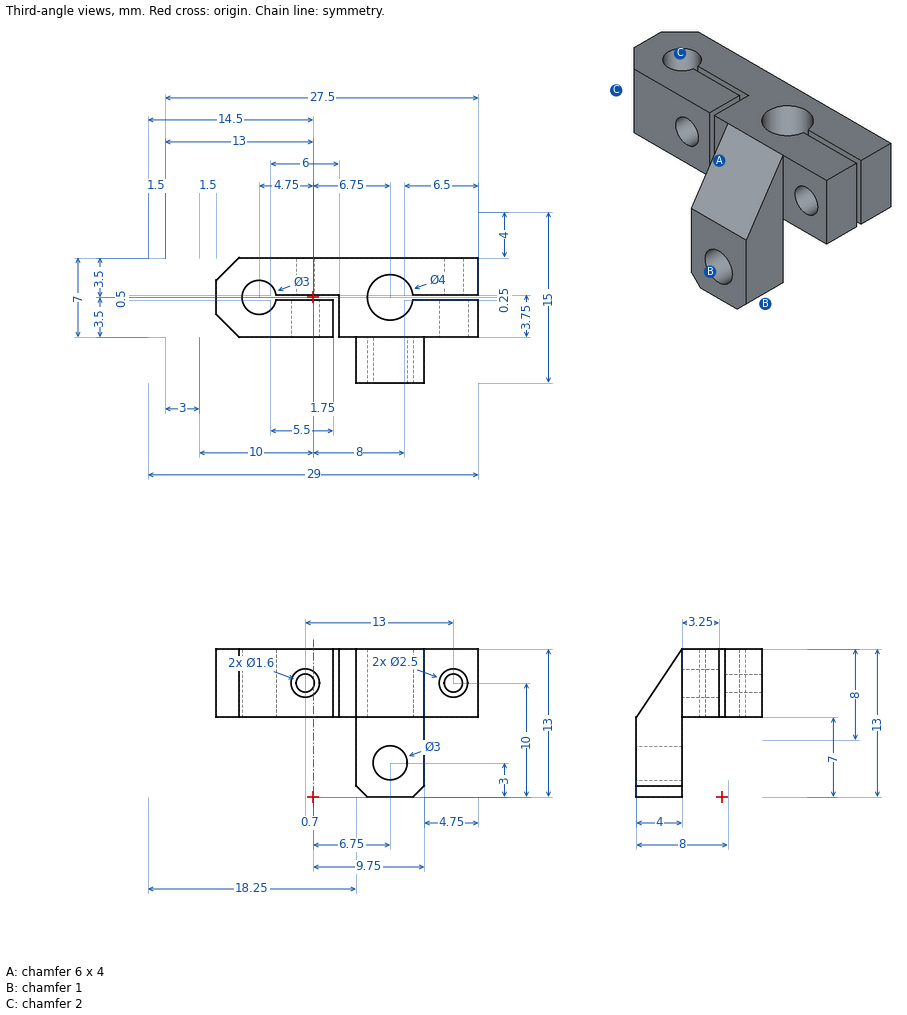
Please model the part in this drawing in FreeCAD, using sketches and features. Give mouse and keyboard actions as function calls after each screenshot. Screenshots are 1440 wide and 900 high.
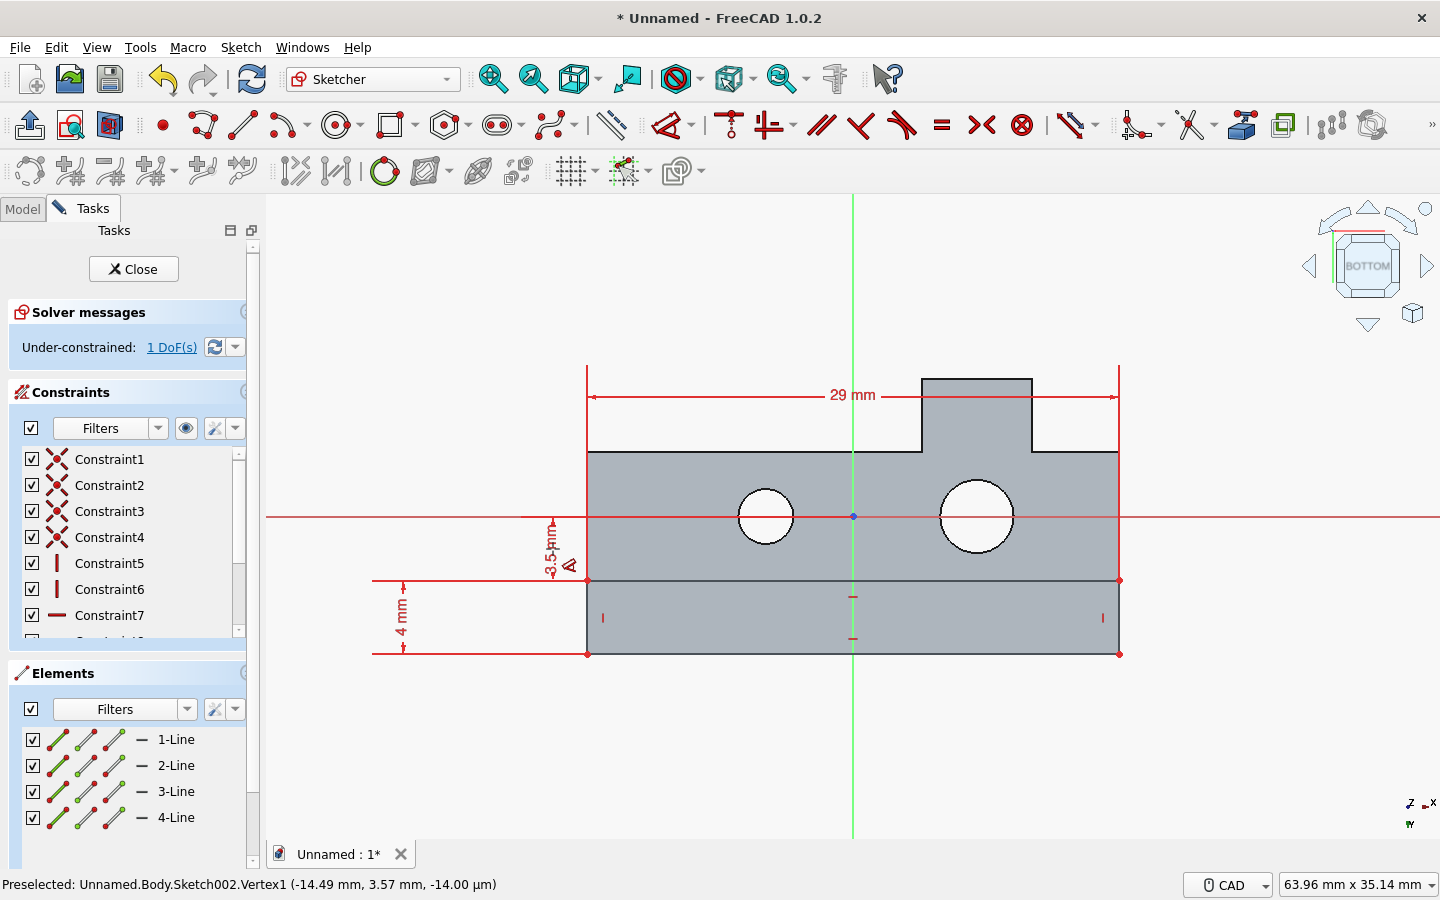
click(587, 581)
click(720, 482)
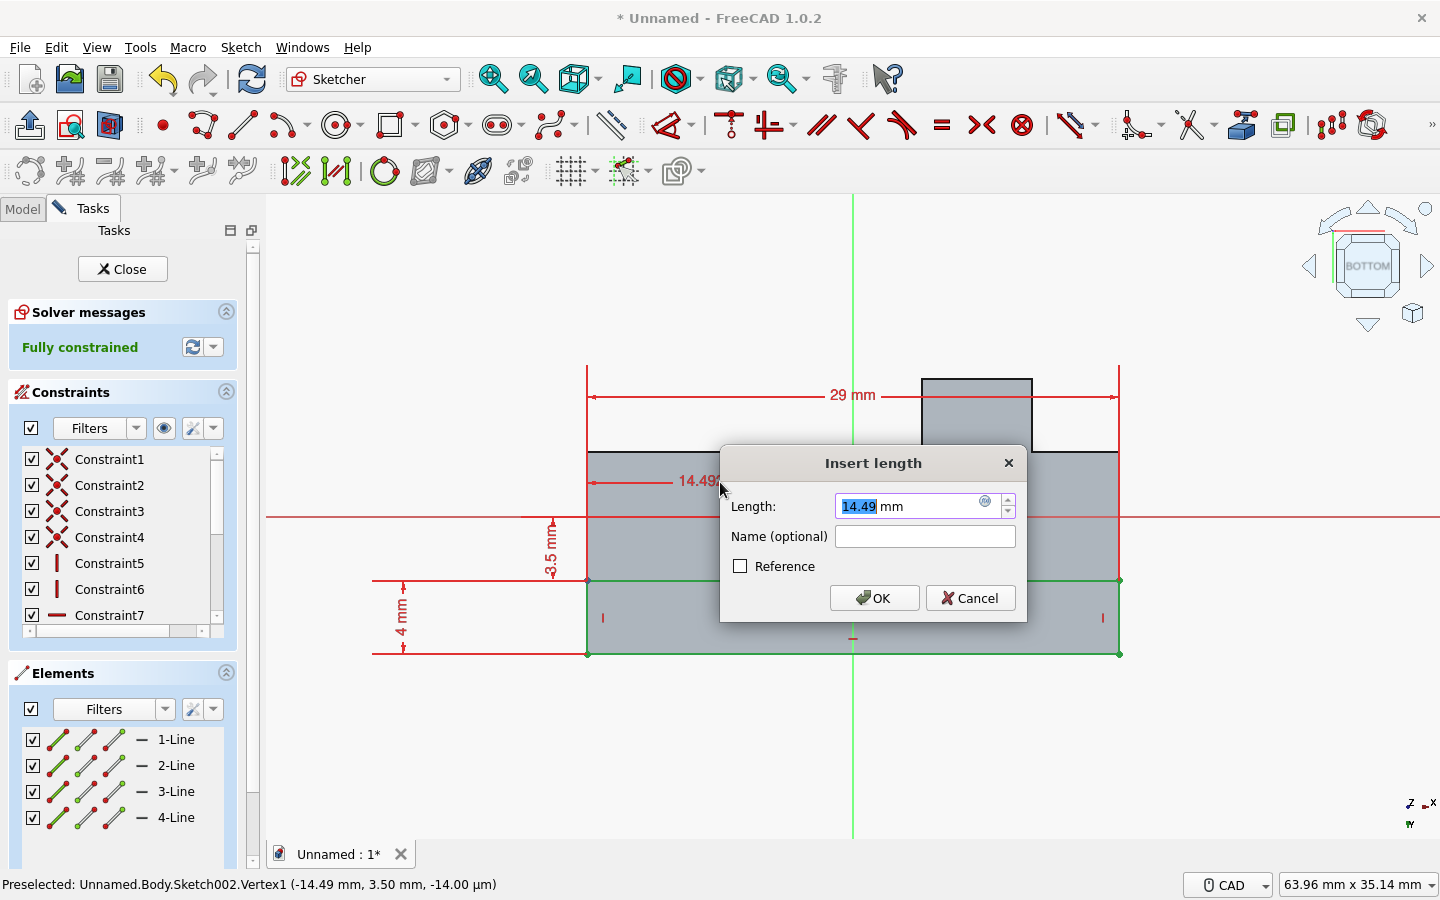
text(14.5)
key(Return)
key(Escape)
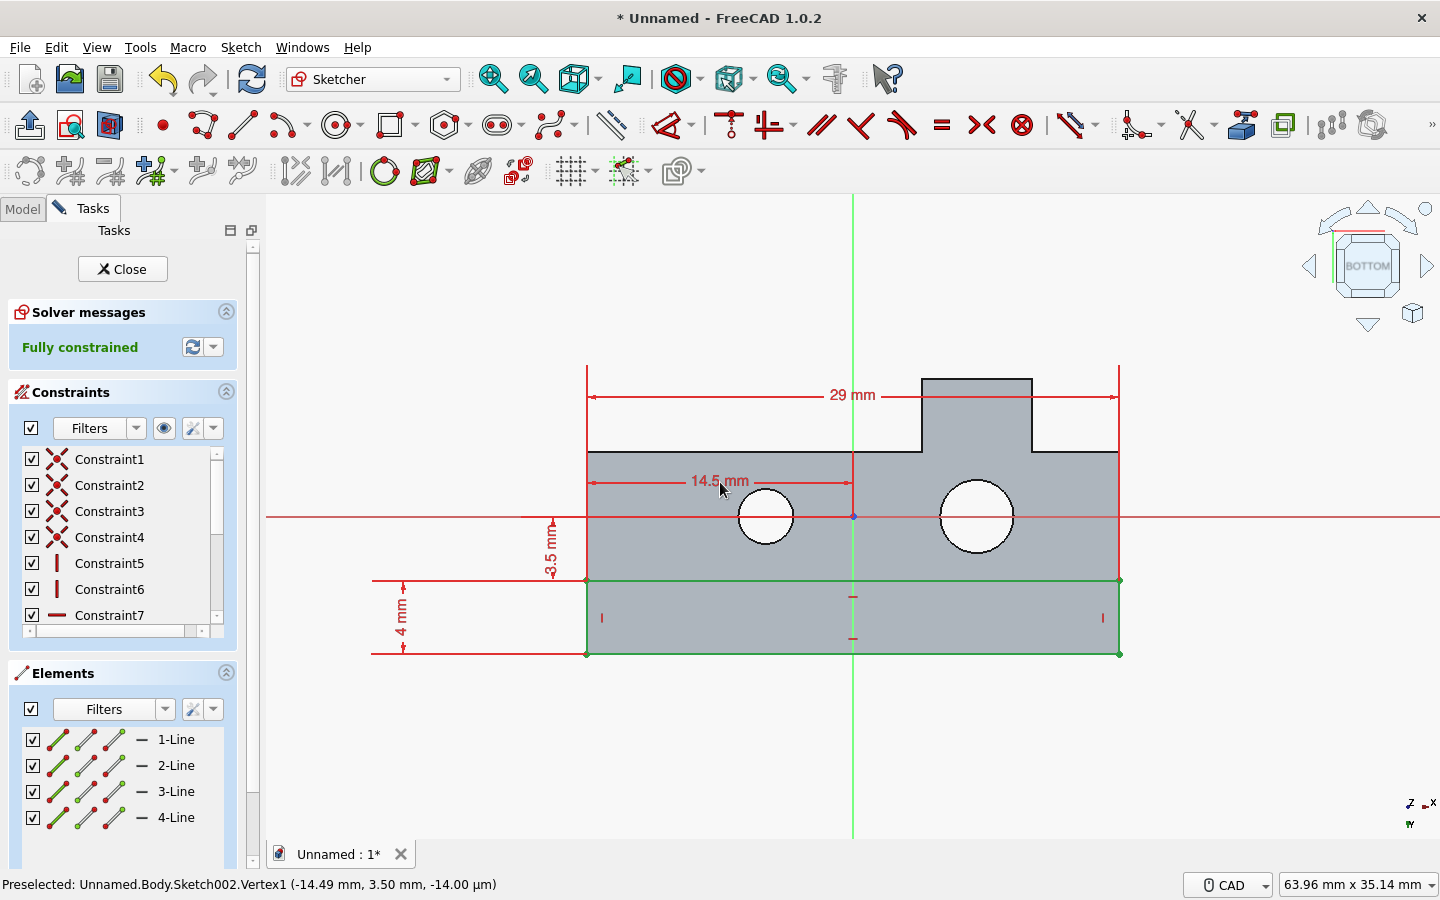
click(123, 269)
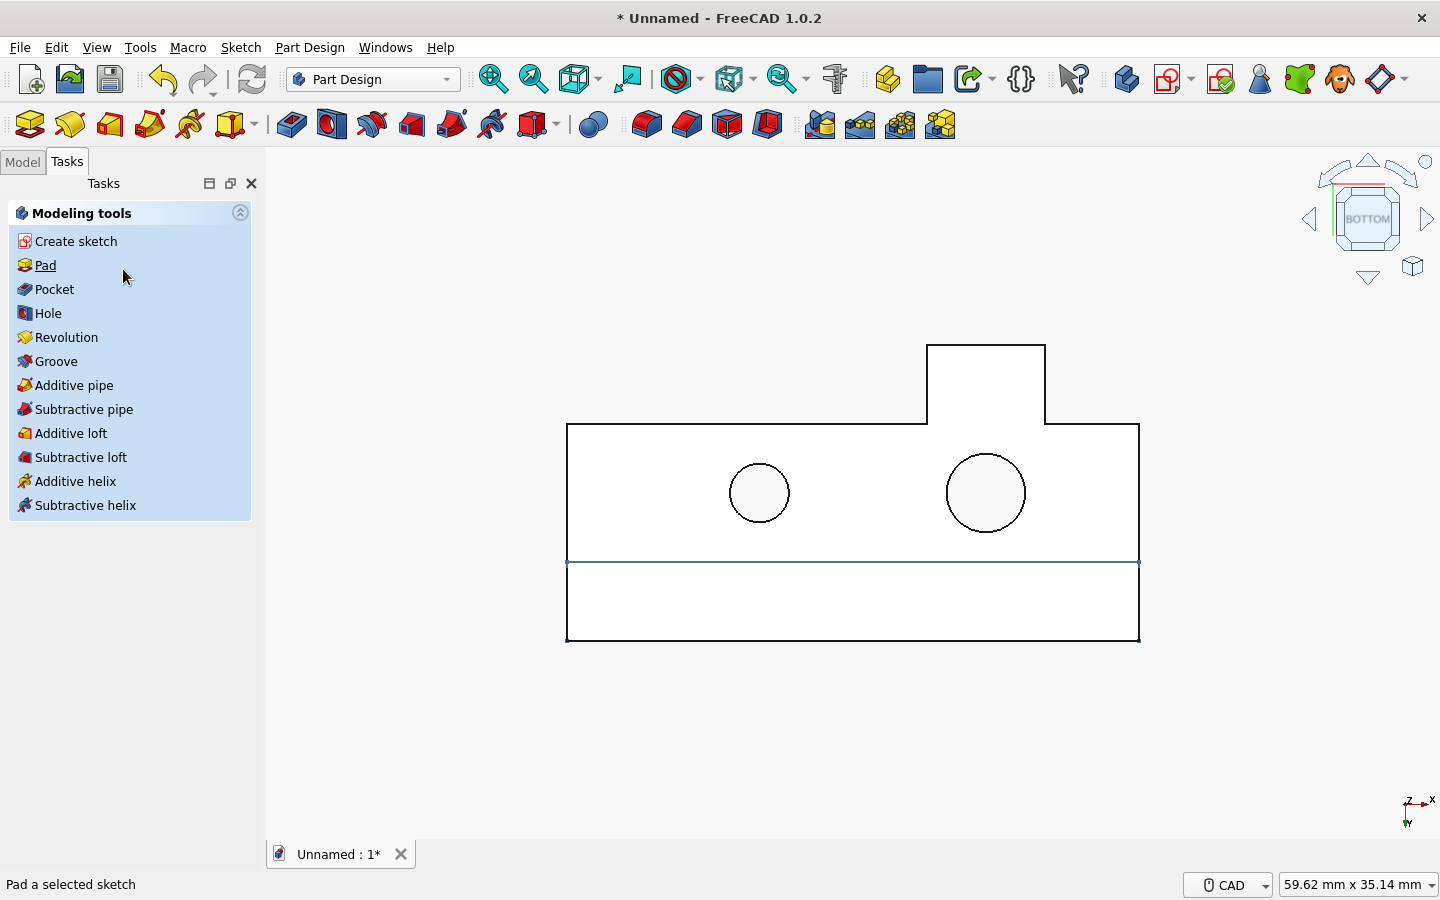
click(292, 124)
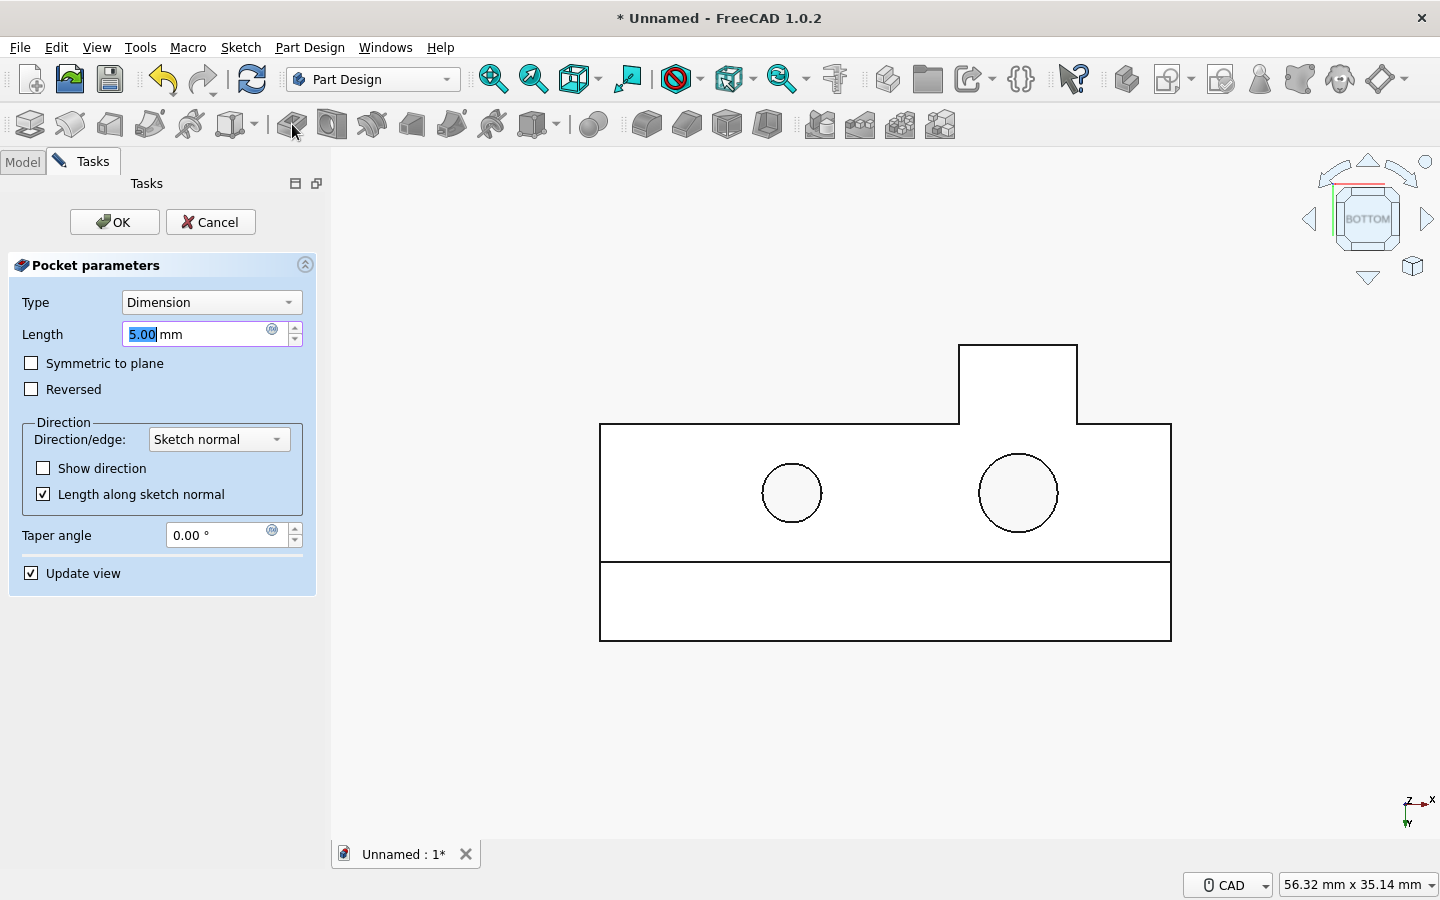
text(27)
key(Tab)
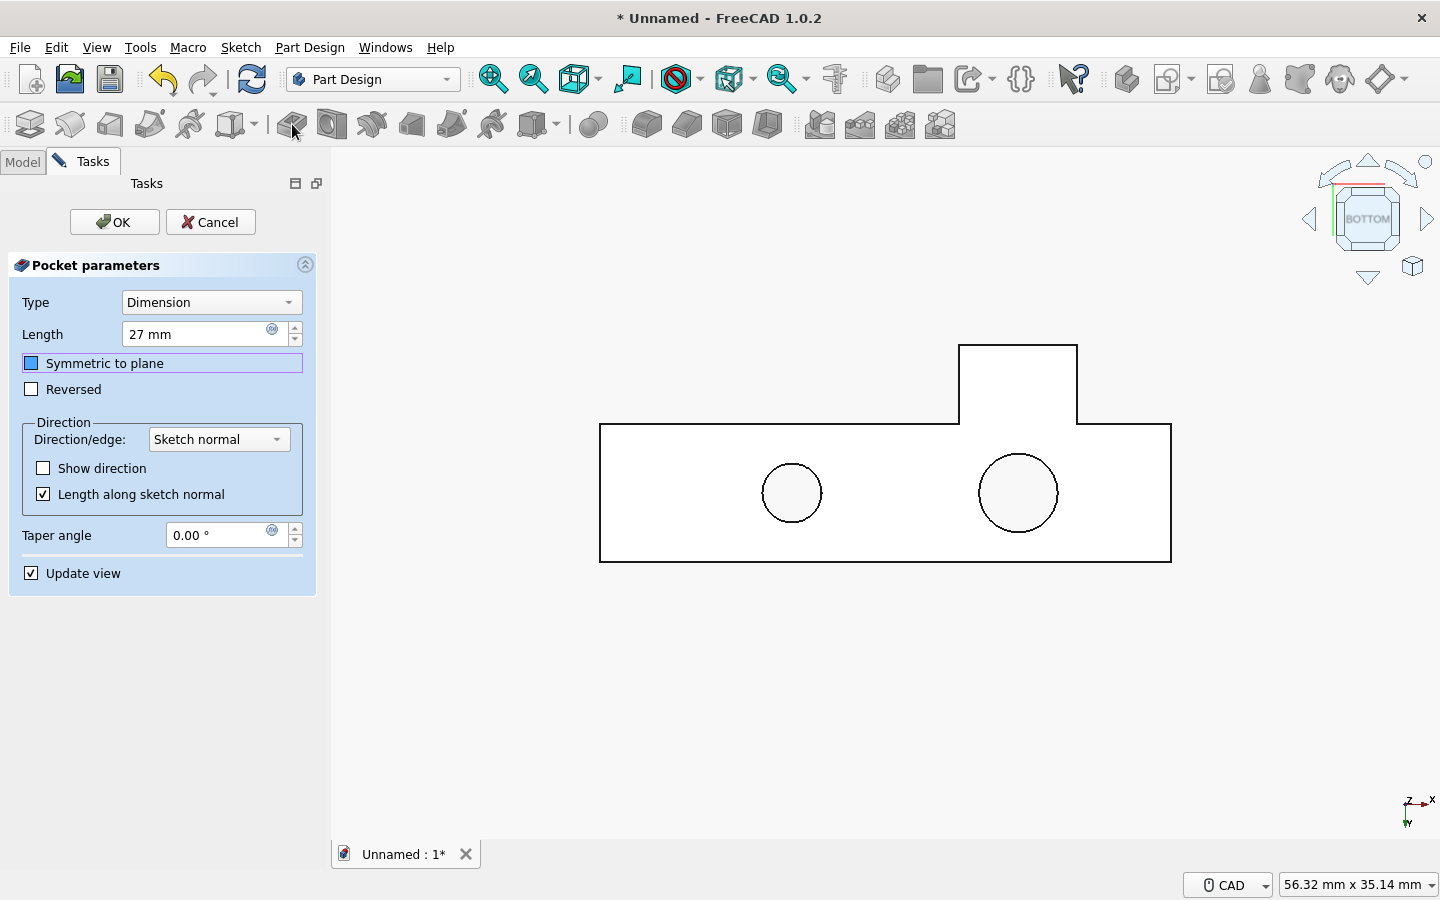
click(115, 222)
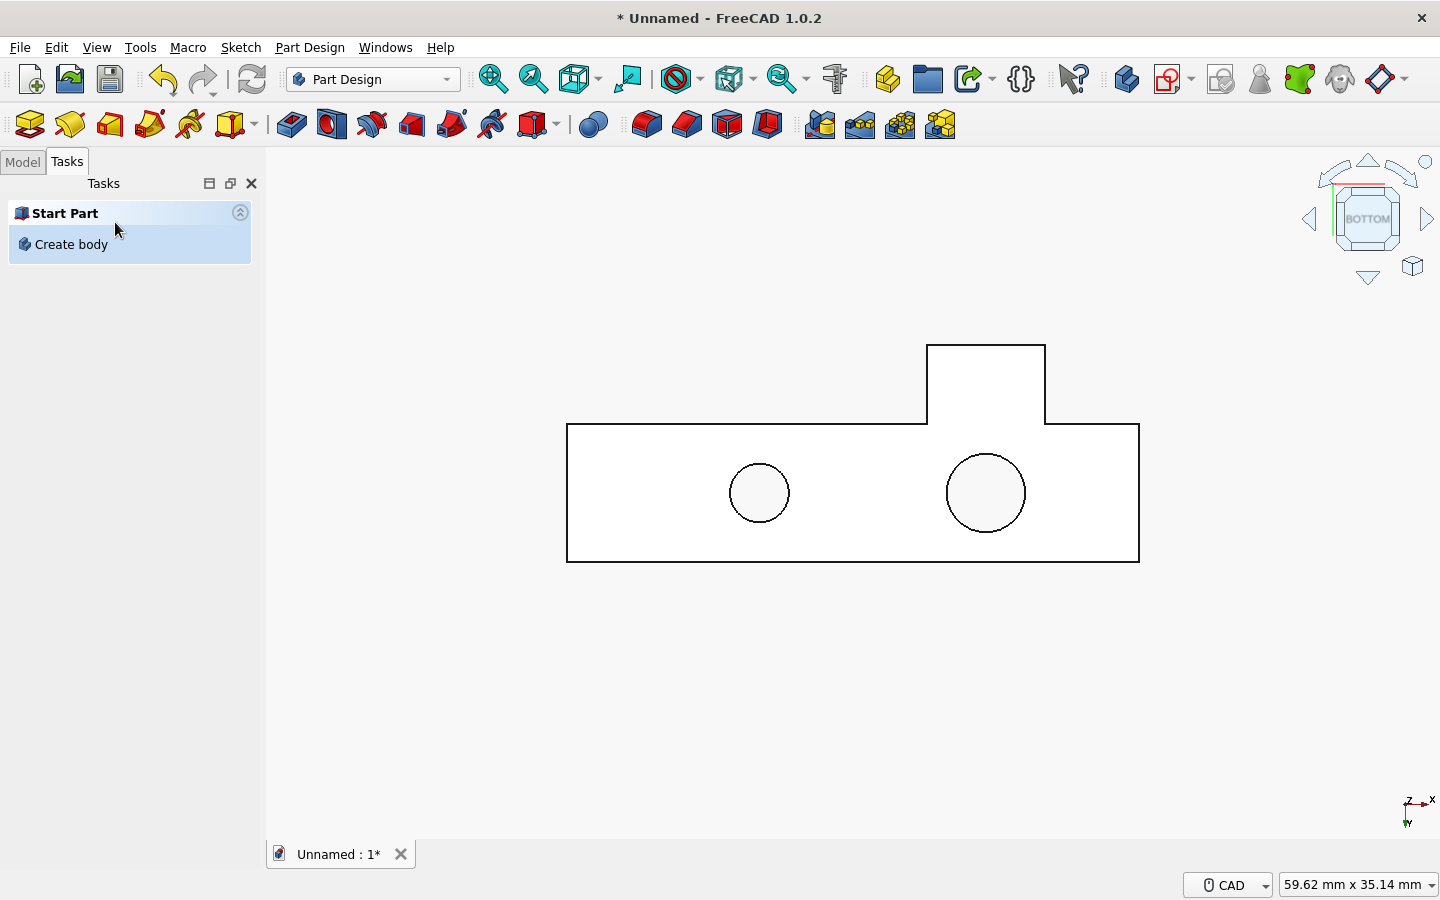
click(853, 484)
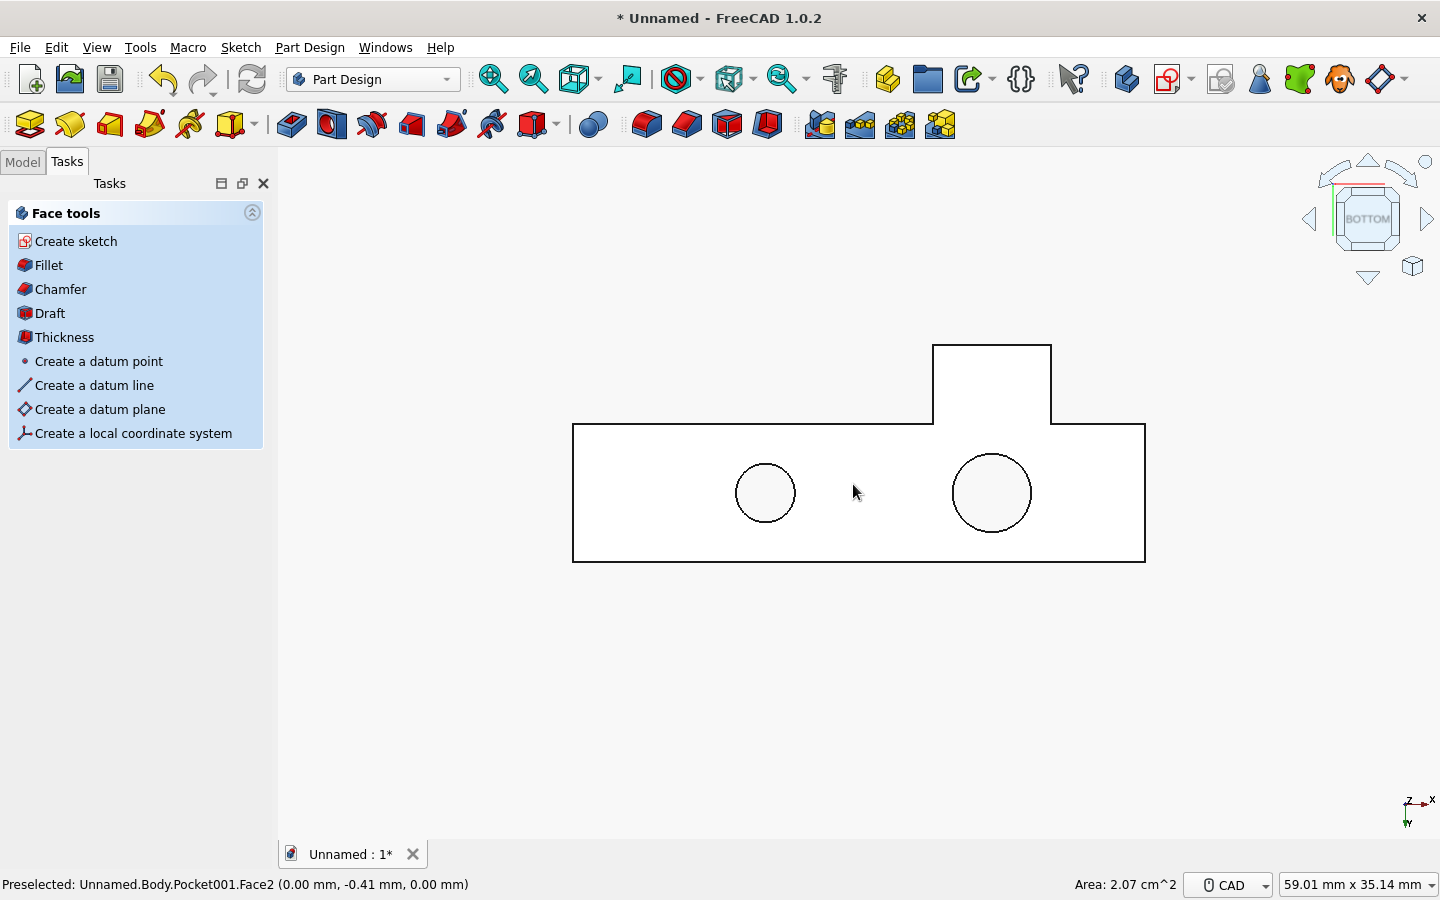
click(1168, 80)